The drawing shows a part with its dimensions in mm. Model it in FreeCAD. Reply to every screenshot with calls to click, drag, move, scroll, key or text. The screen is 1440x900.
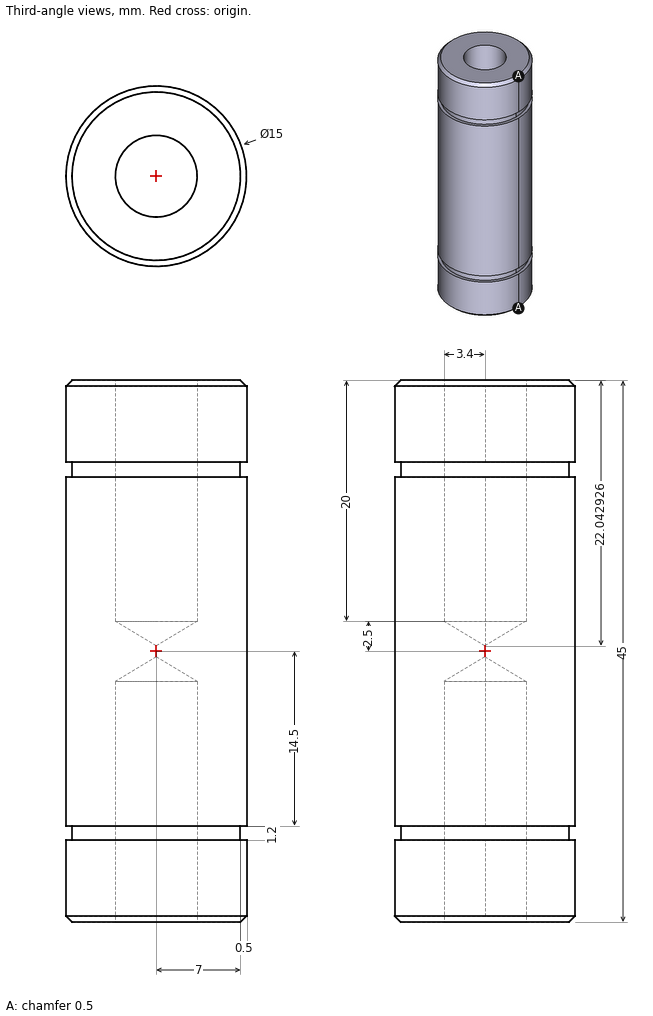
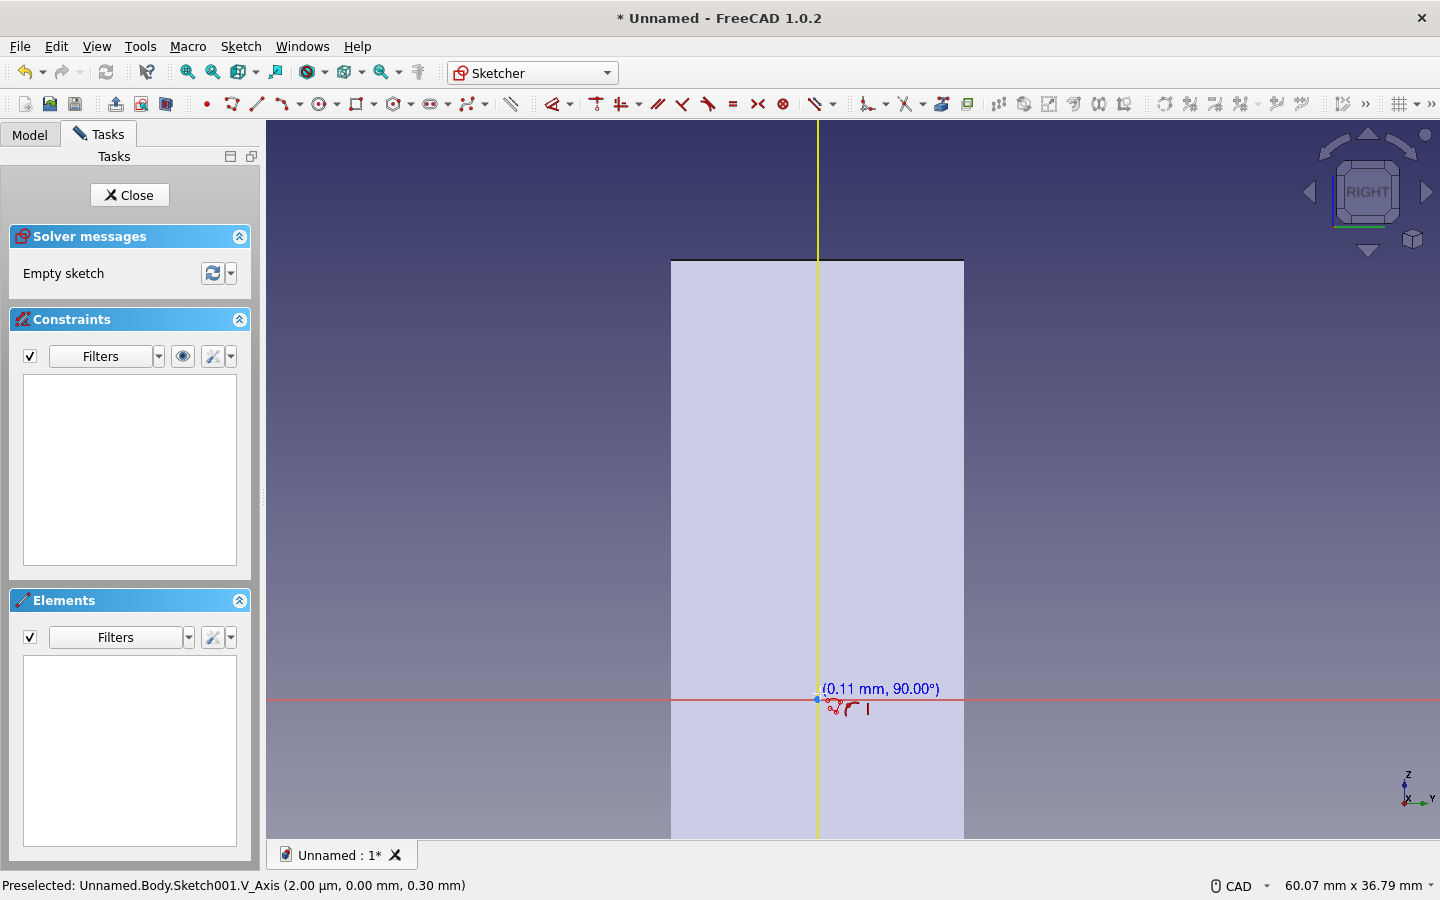
click(809, 260)
click(751, 260)
click(751, 651)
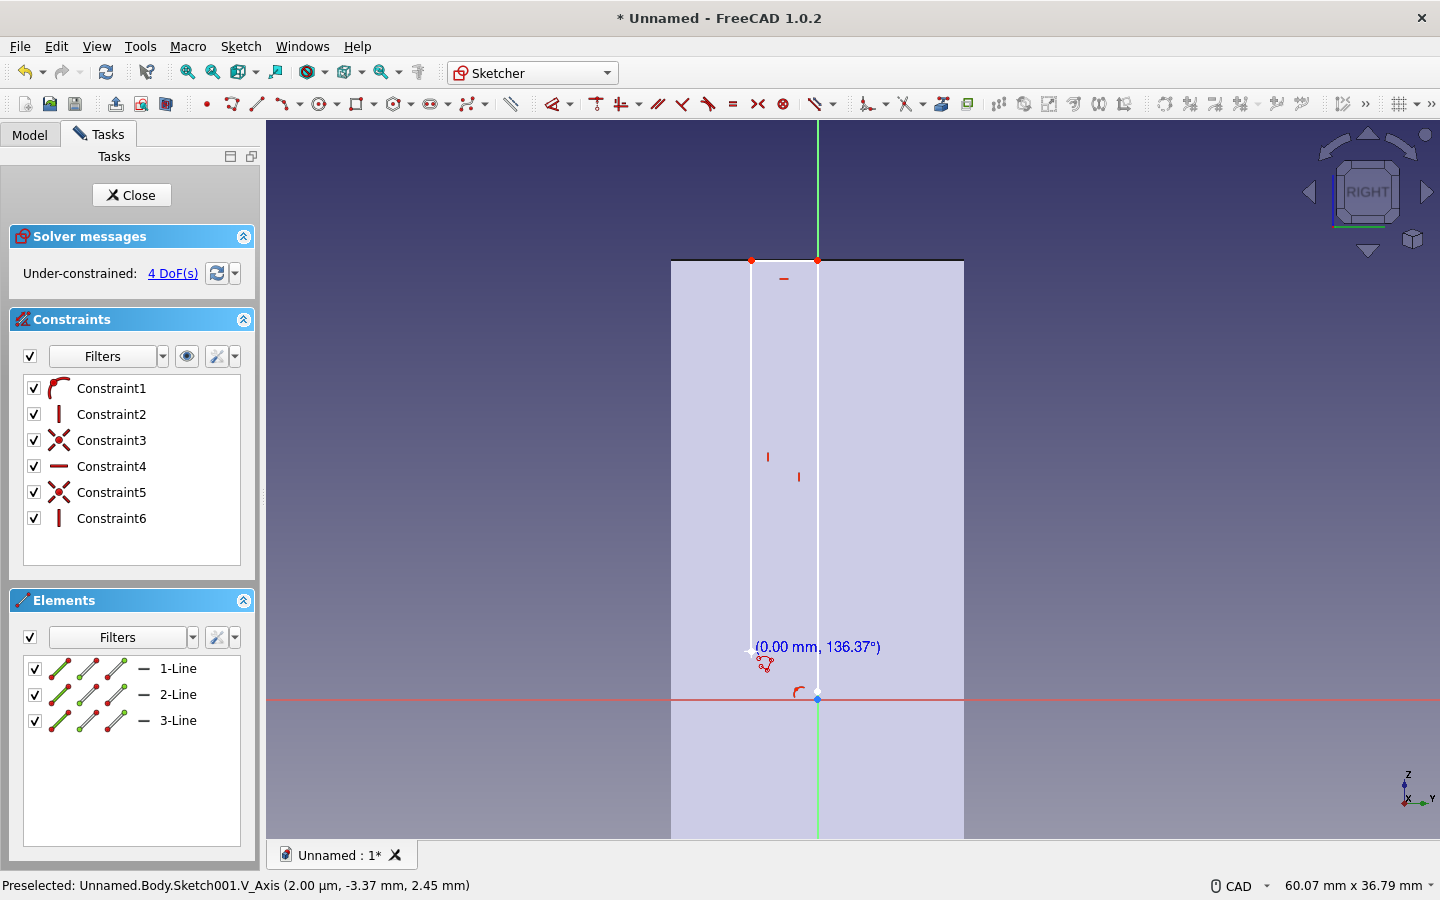
scroll(818, 691, up, 3)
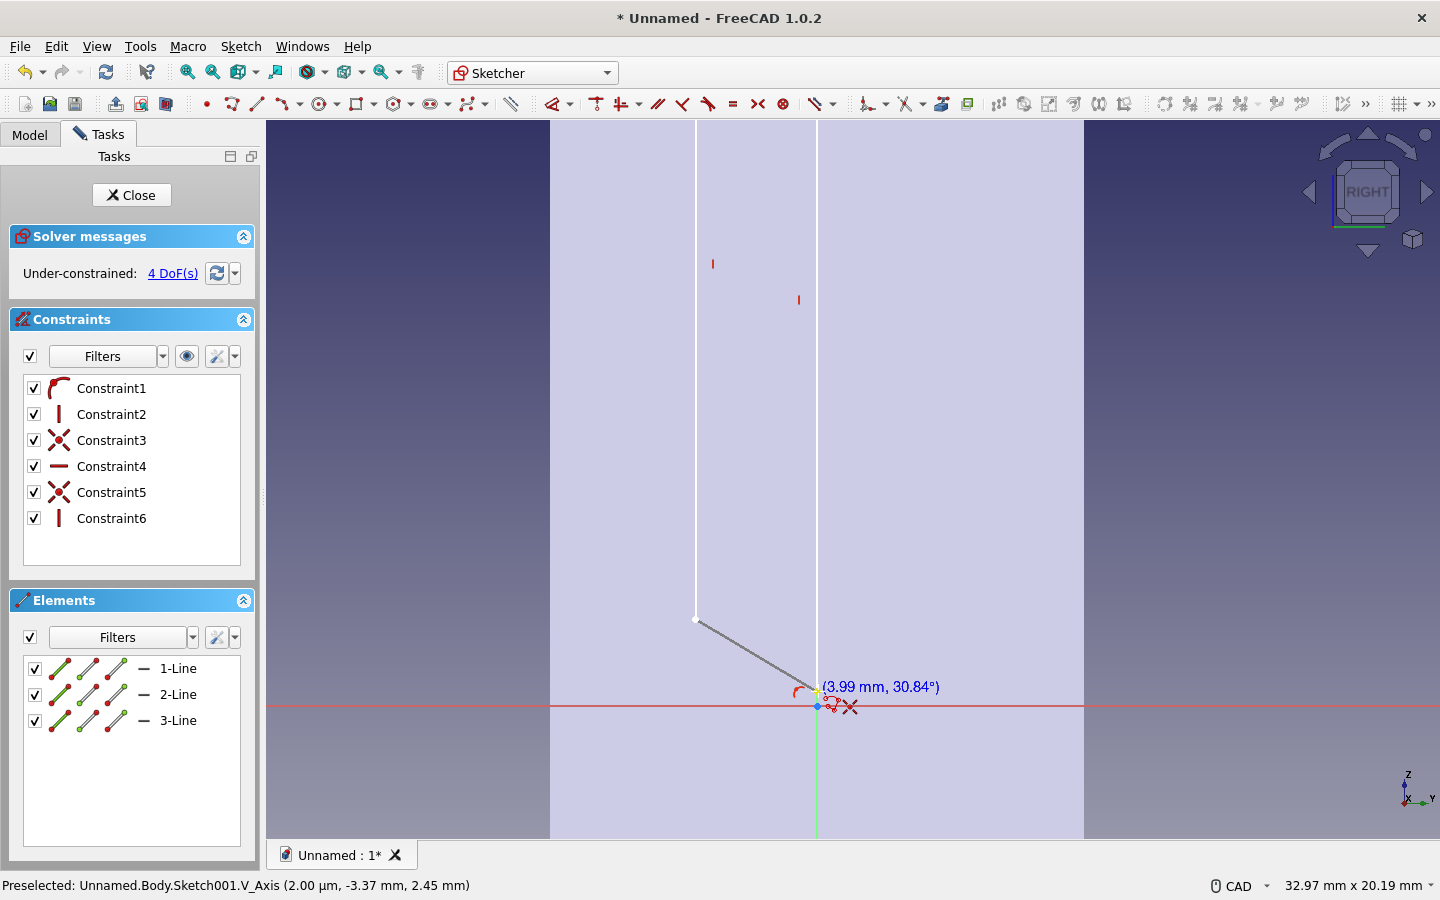
click(817, 692)
key(Escape)
key(Escape)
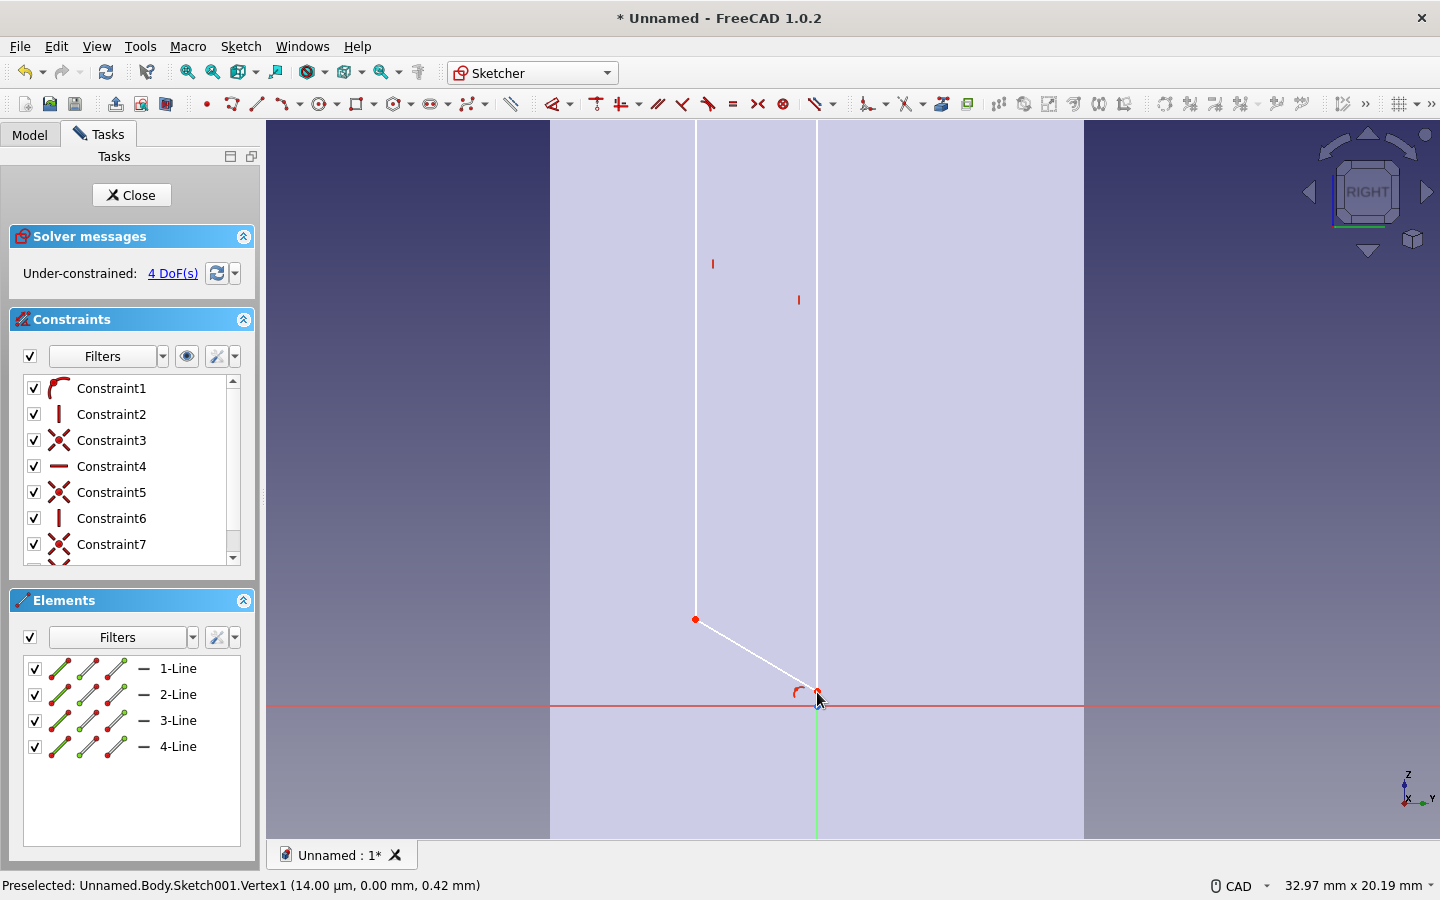
click(696, 406)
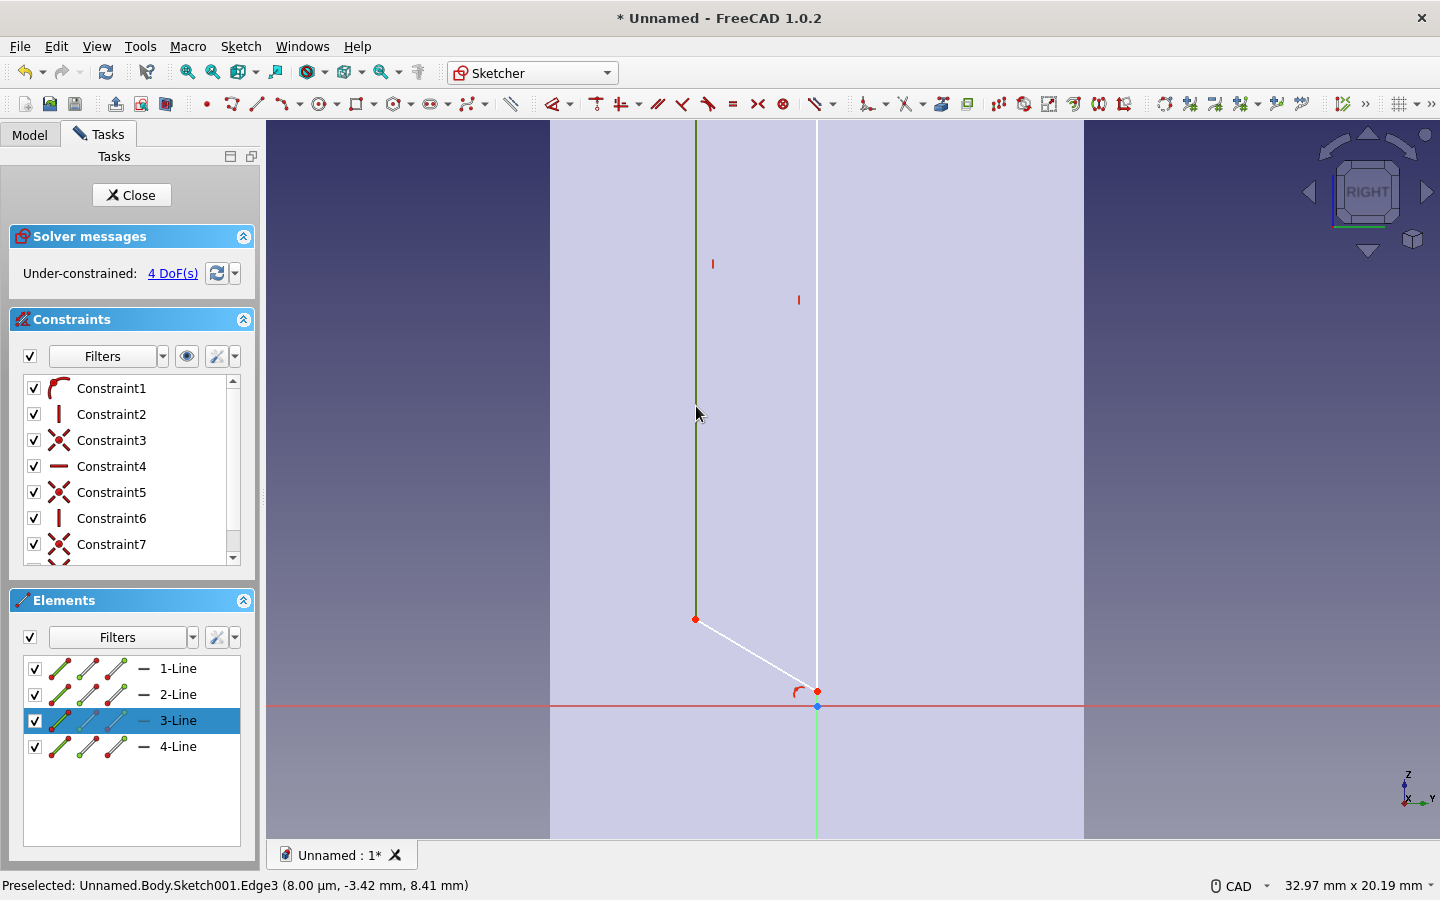
key(i)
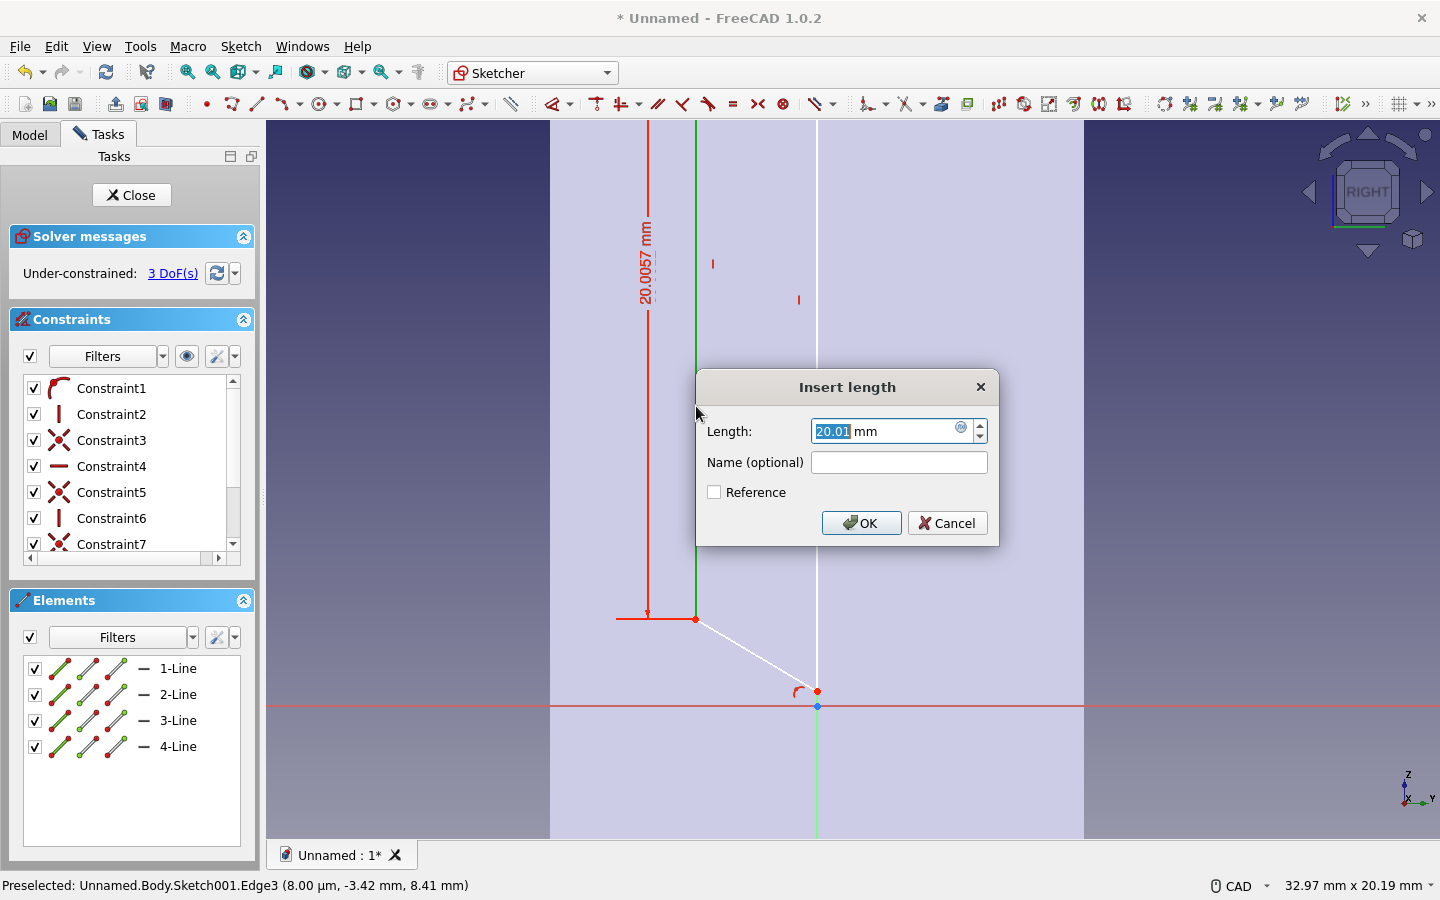
text(20)
key(Return)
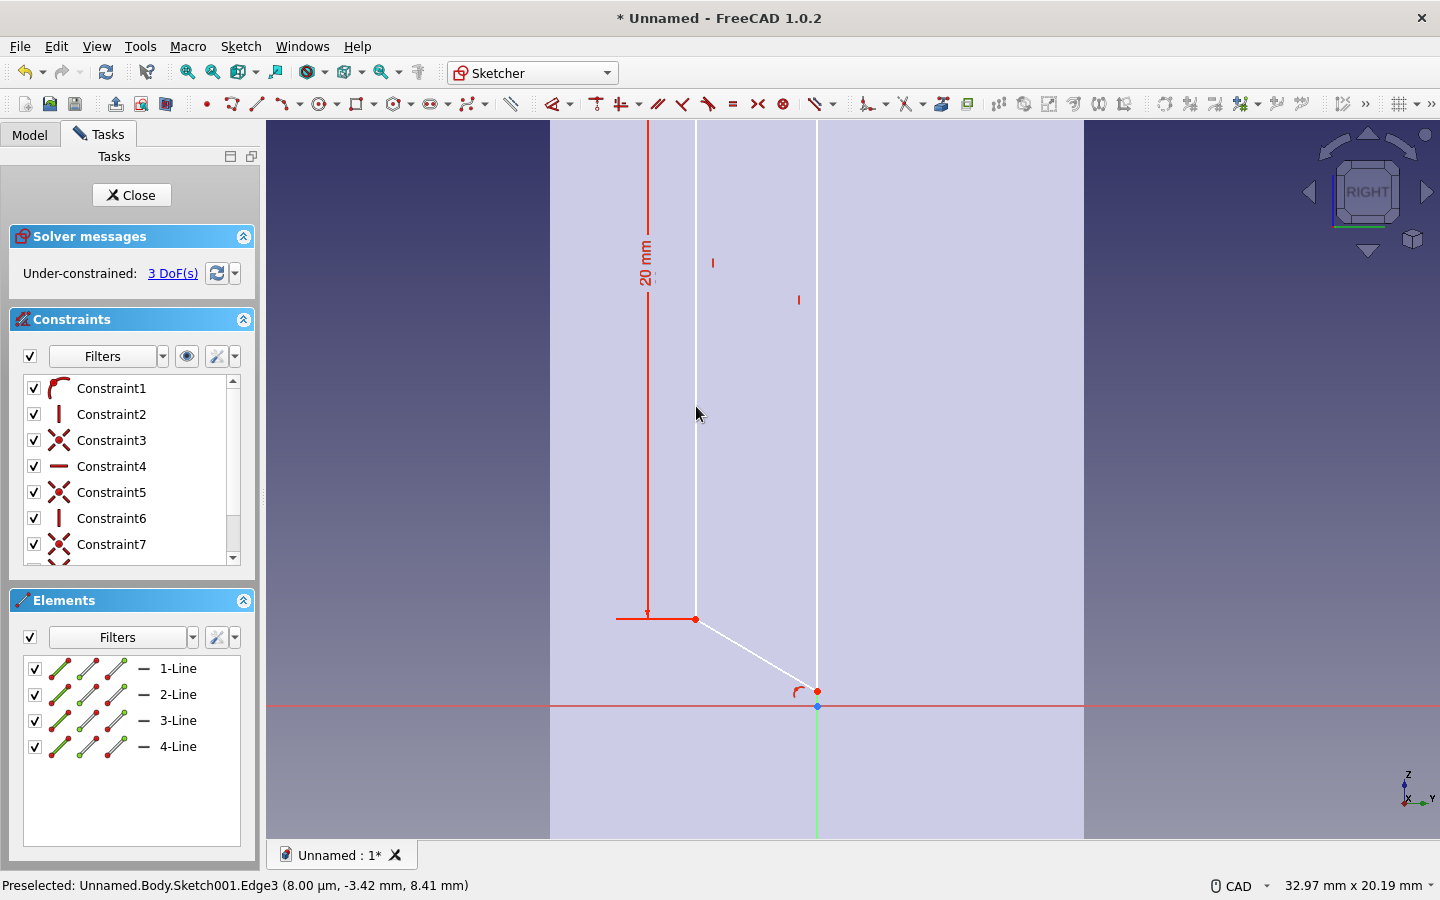
scroll(818, 691, down, 3)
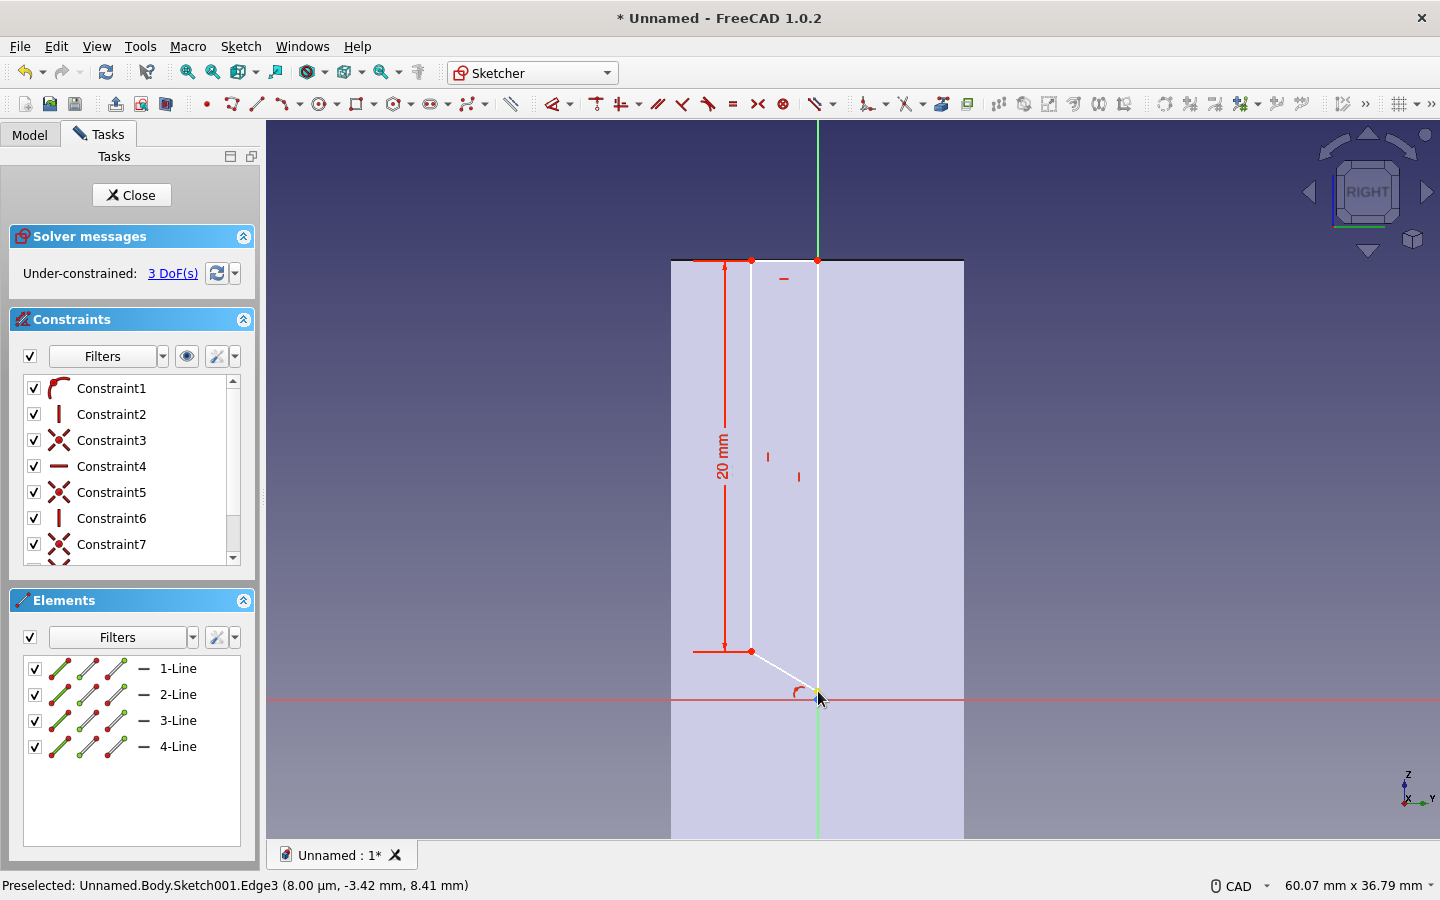
click(798, 261)